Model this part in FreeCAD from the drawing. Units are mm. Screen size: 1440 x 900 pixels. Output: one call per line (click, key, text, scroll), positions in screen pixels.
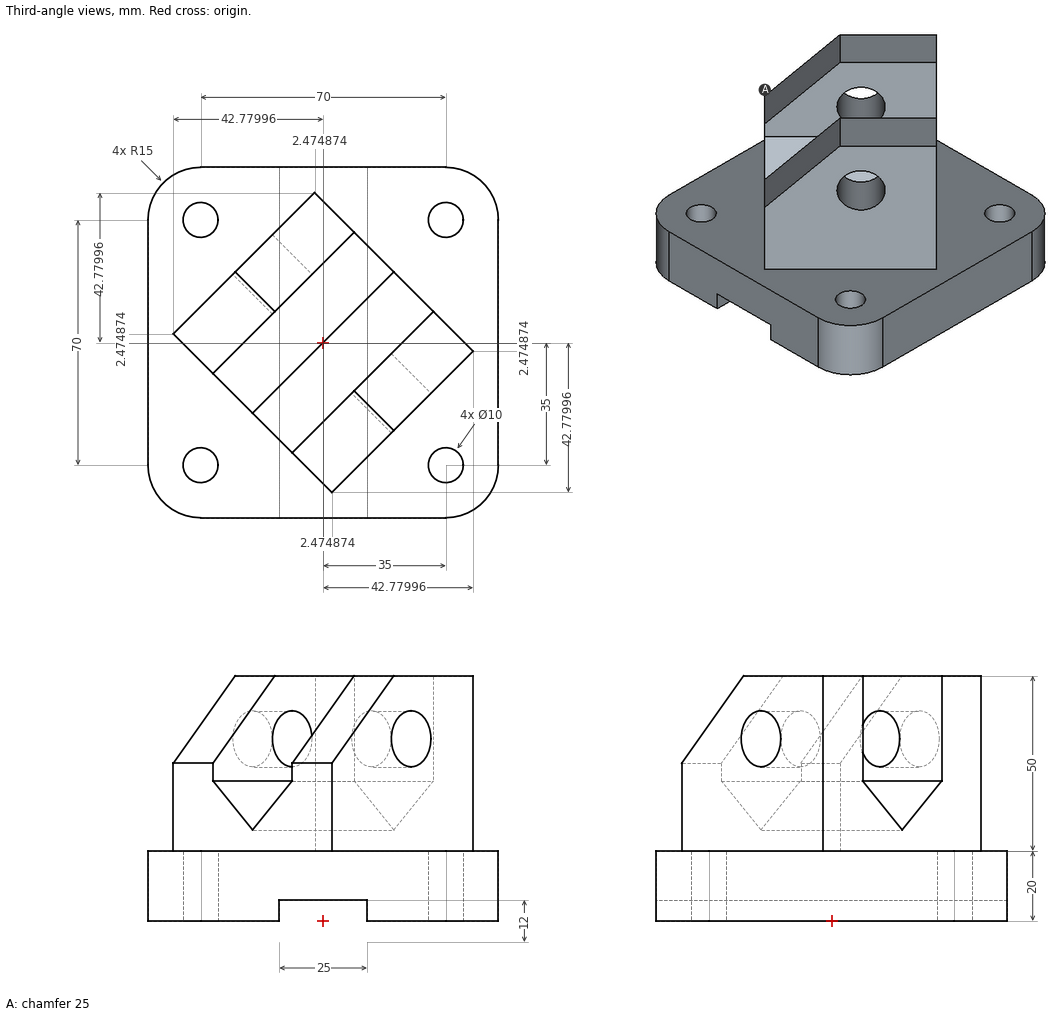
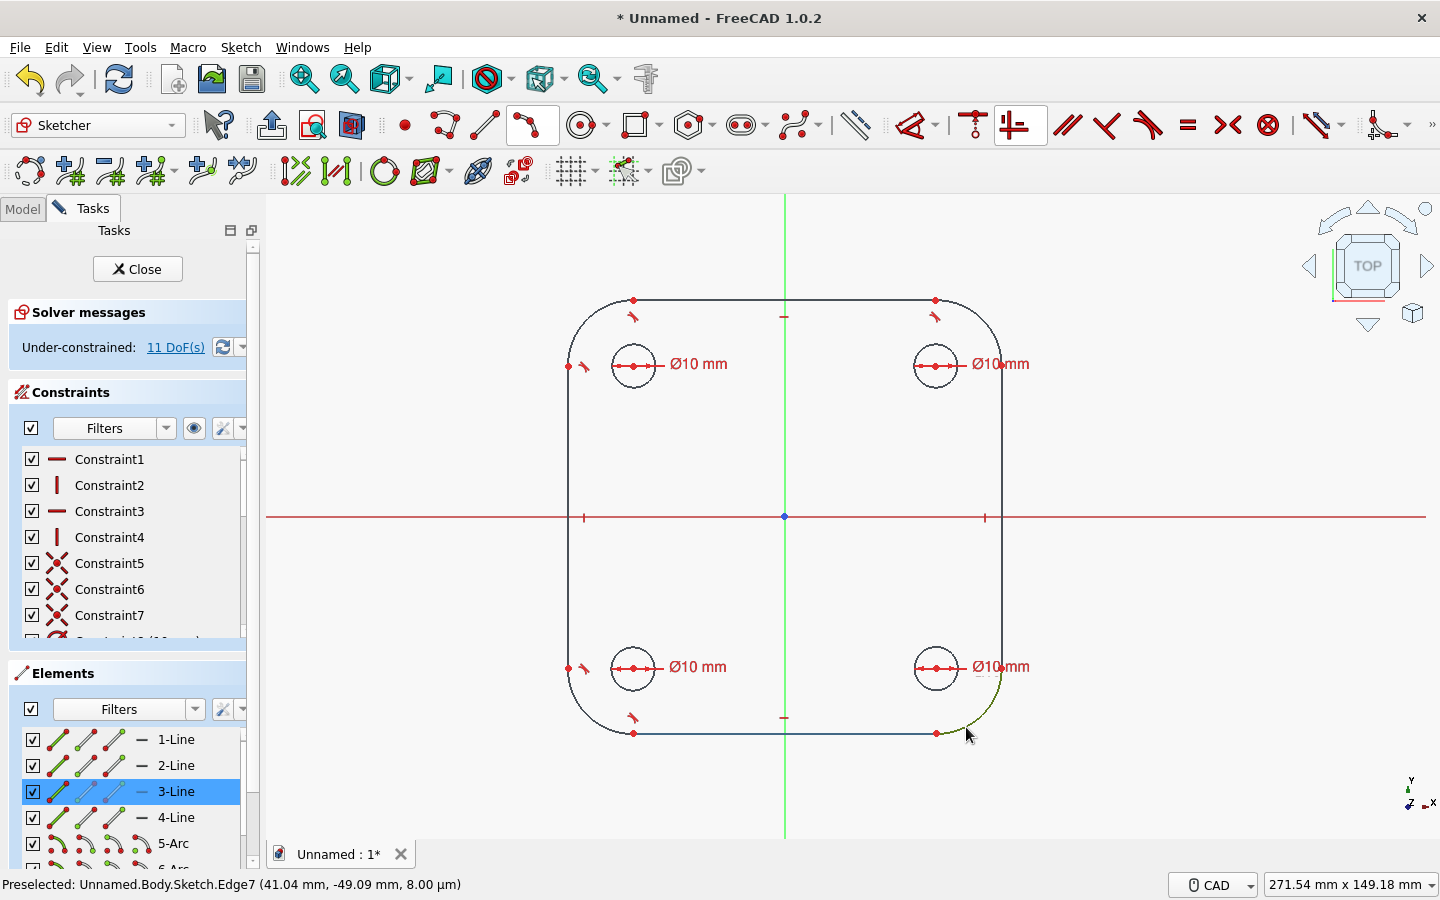
key(t)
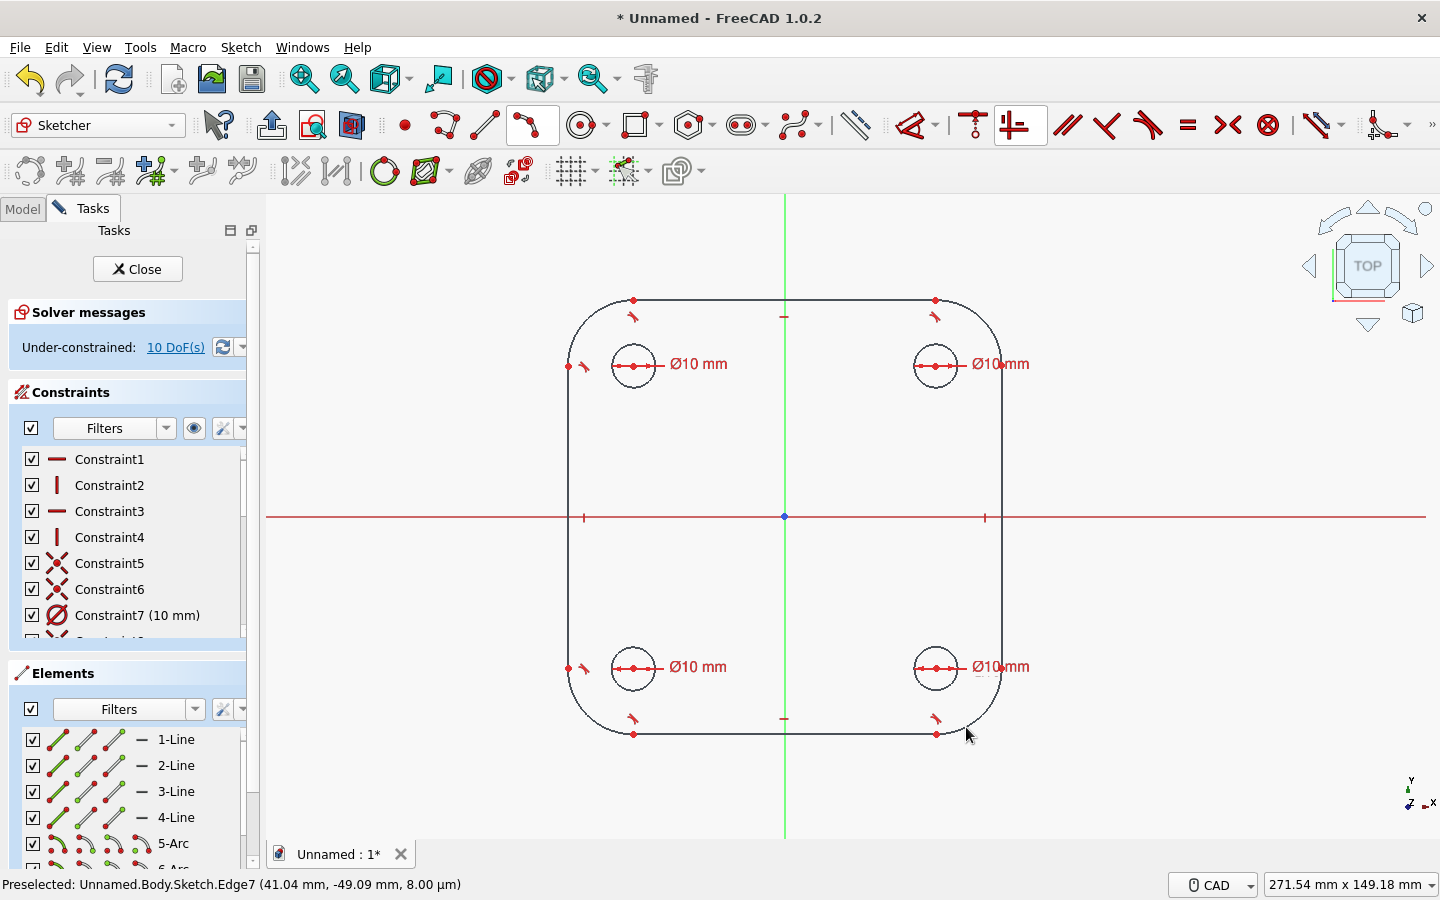
click(1002, 578)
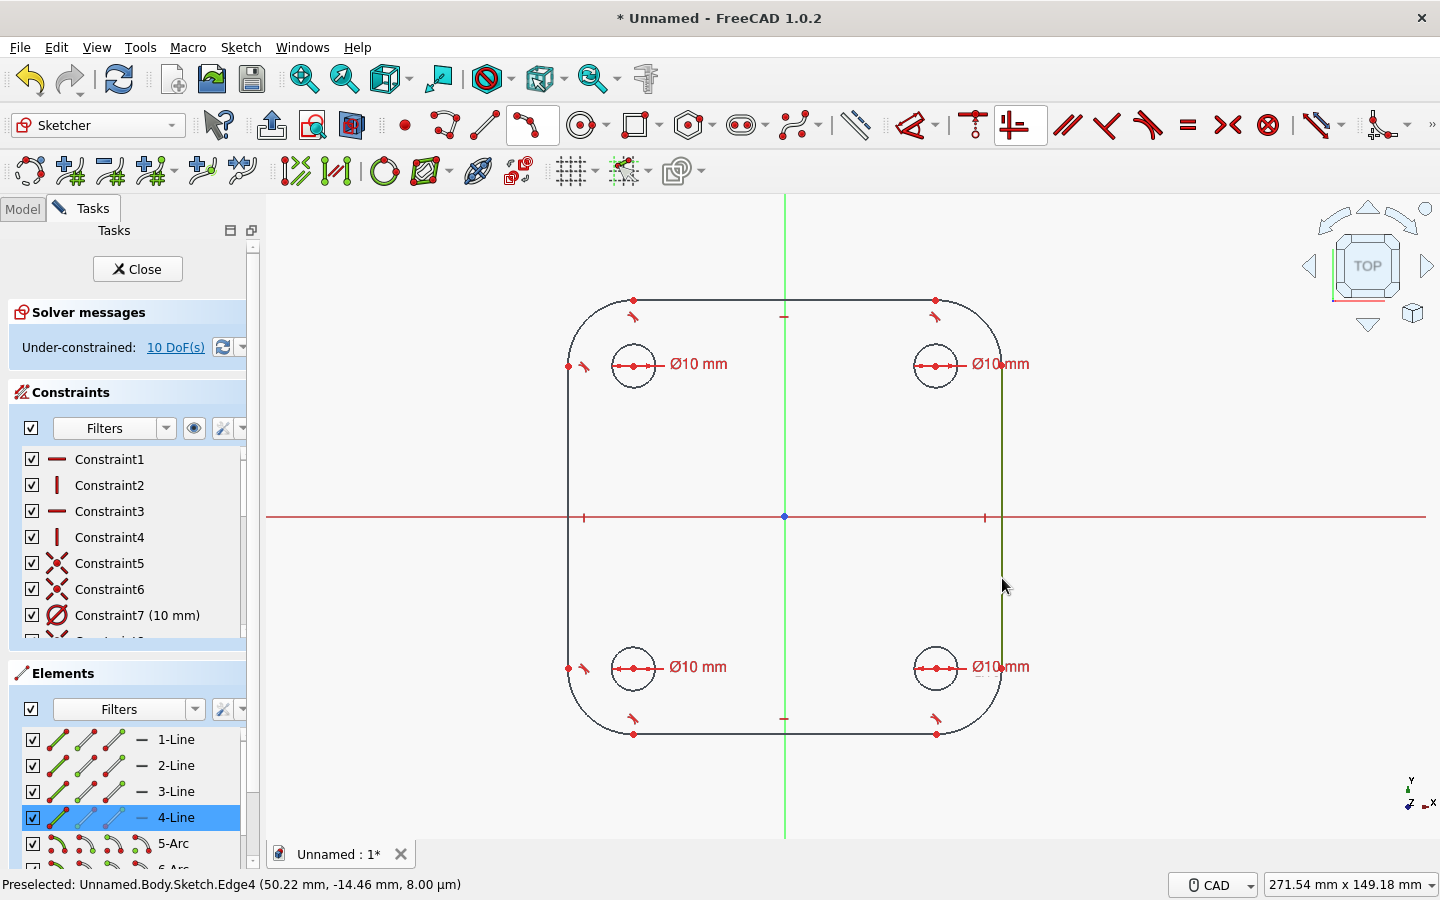
click(966, 727)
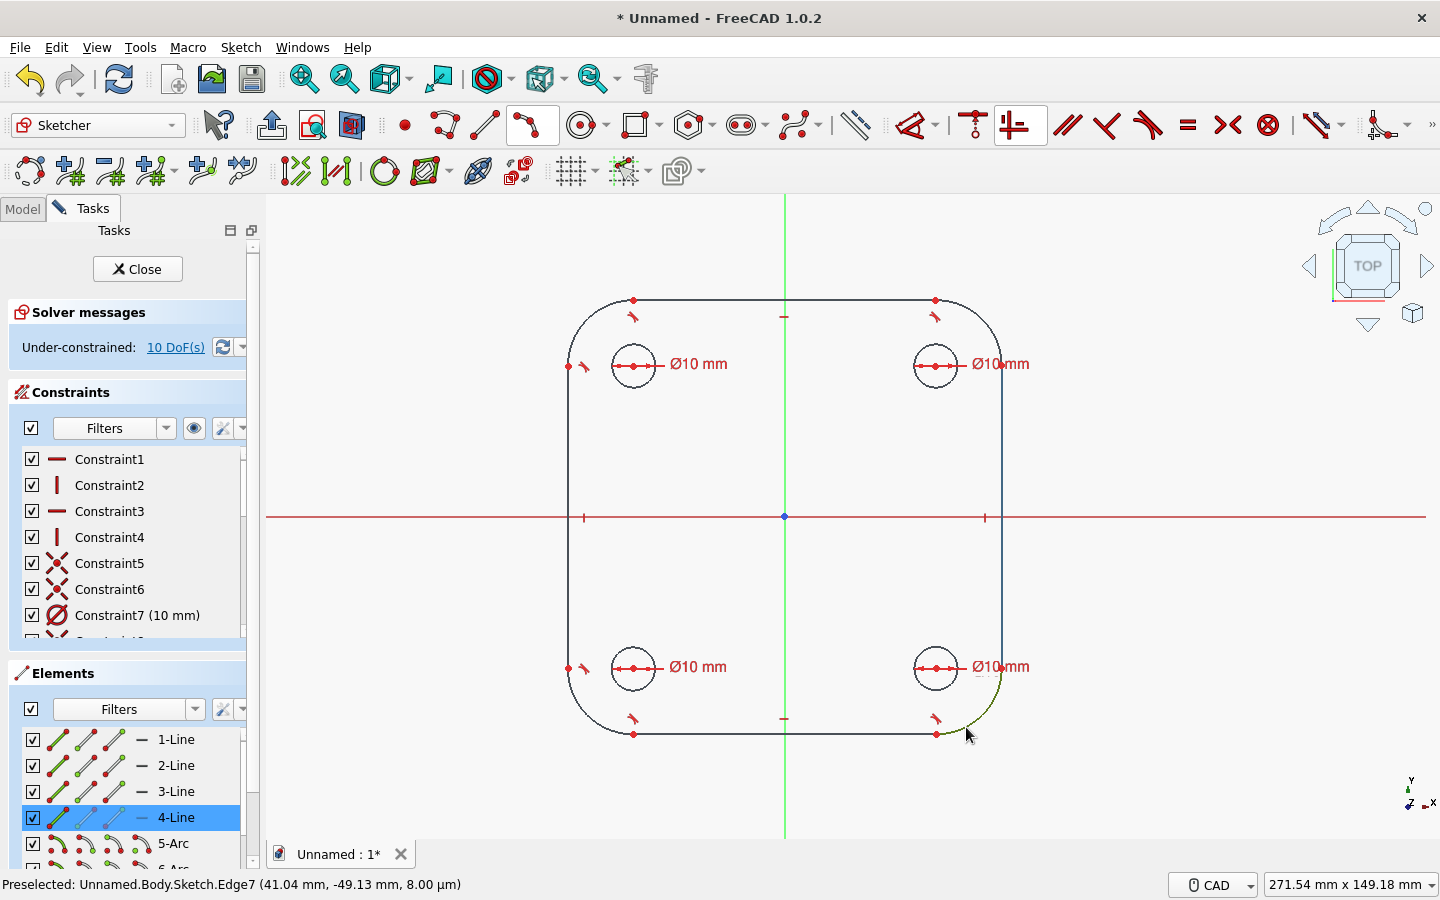
key(t)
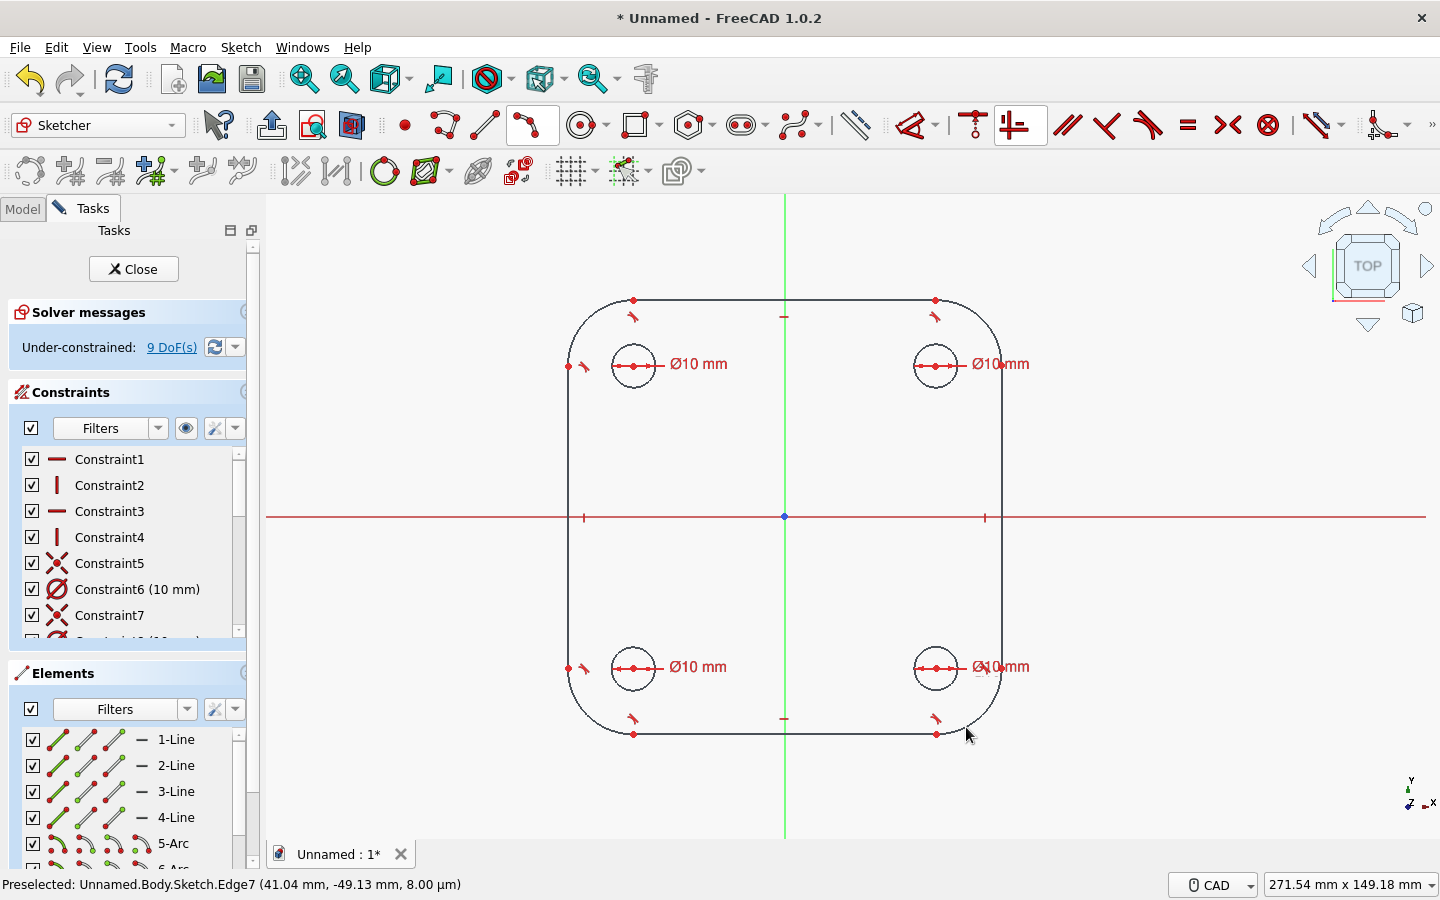
click(1002, 578)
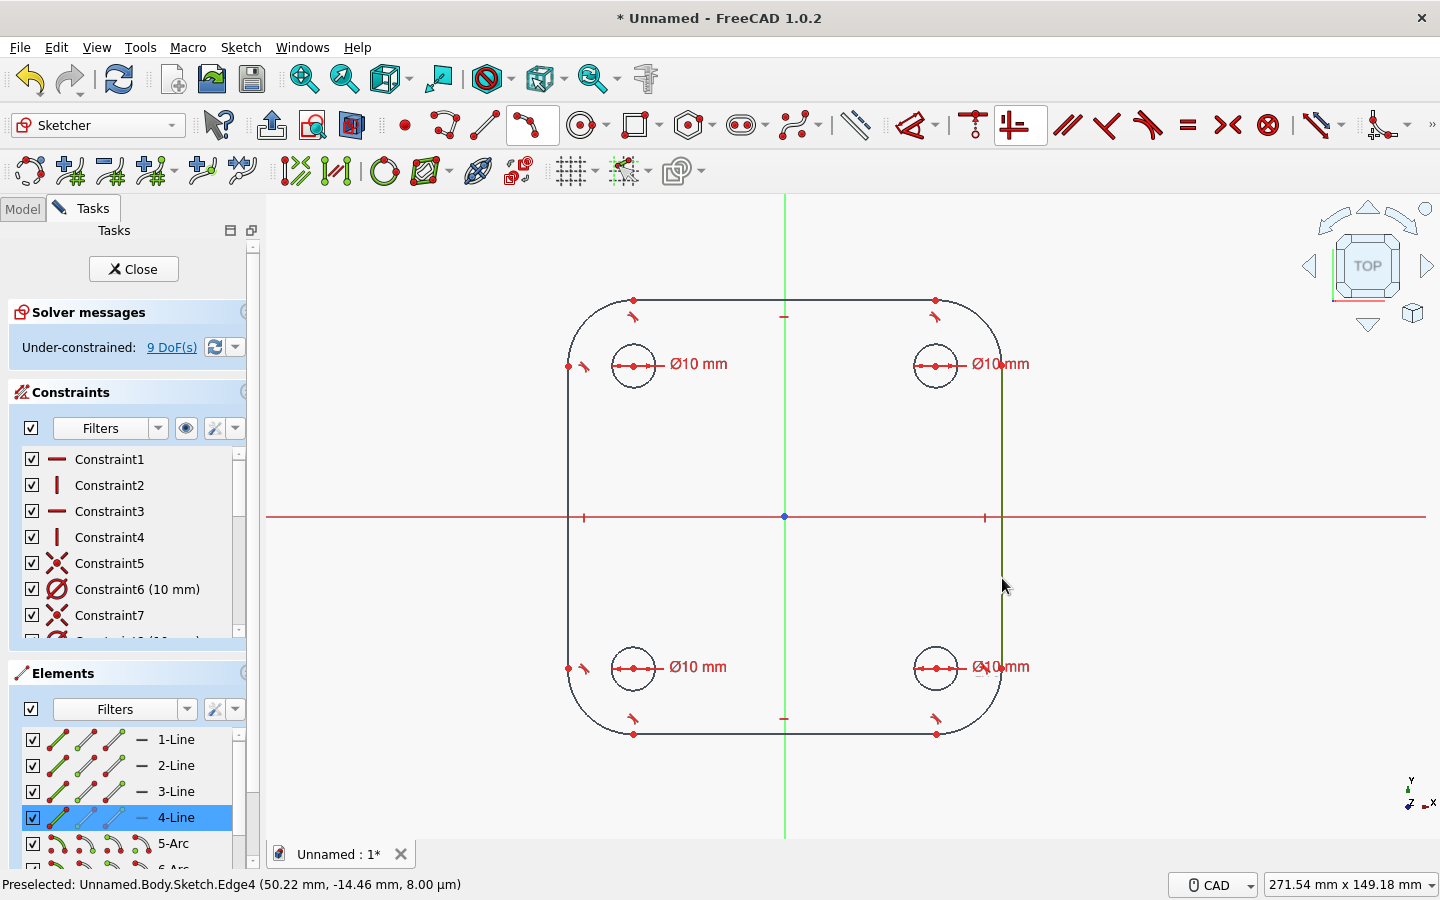
click(994, 336)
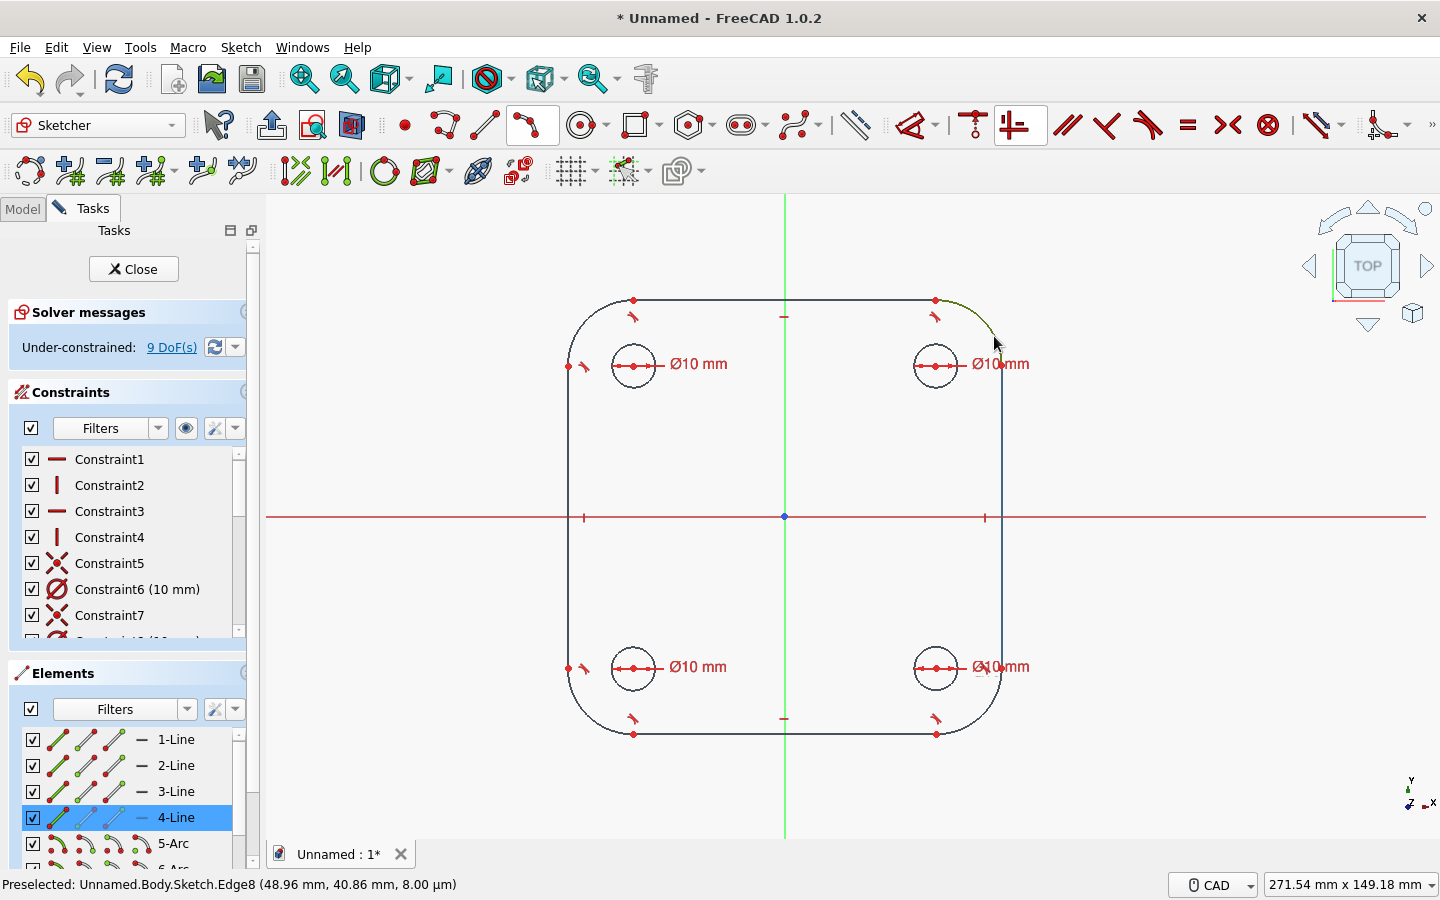
key(t)